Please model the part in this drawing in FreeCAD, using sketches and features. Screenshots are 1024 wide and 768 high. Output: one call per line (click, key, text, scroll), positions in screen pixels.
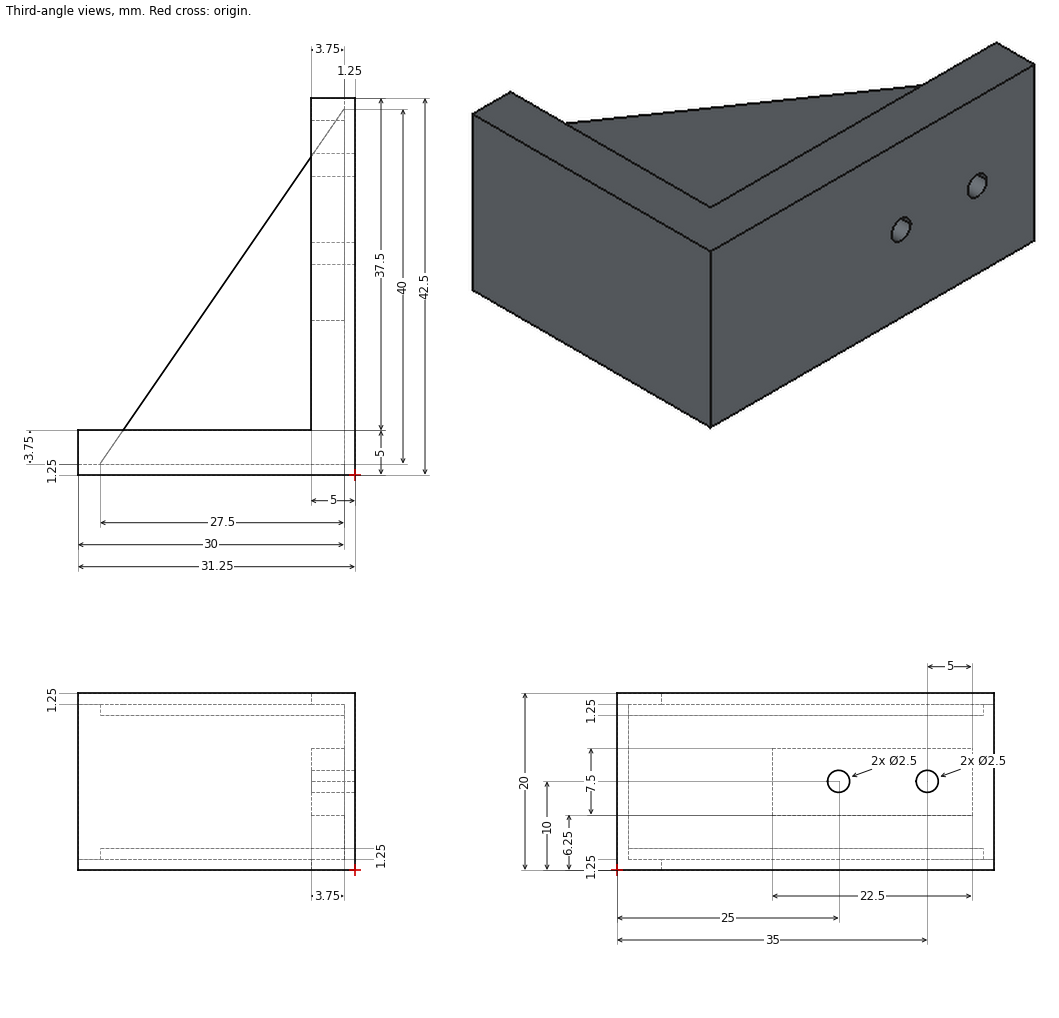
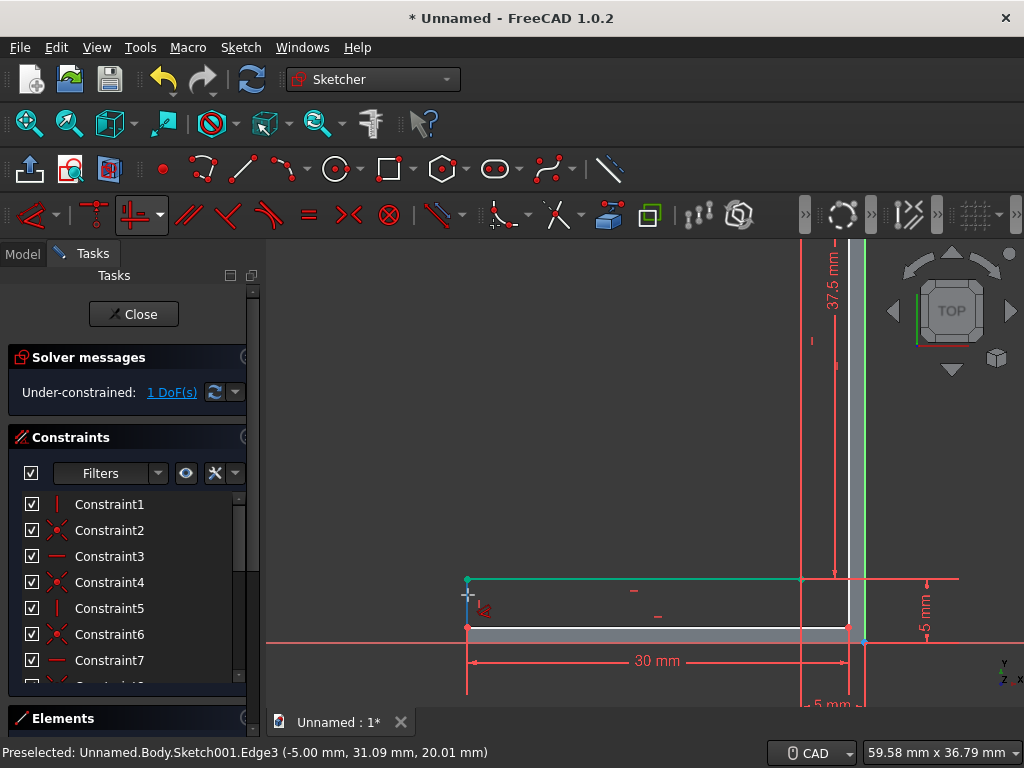
click(467, 594)
click(433, 604)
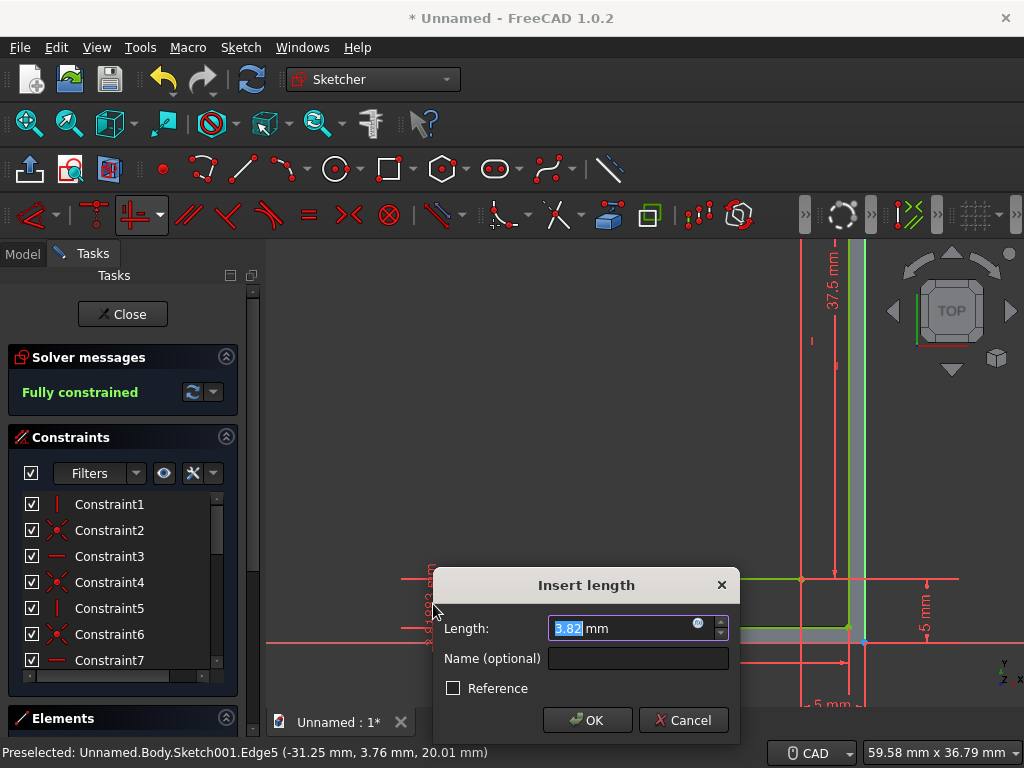
text(3.75)
key(Return)
key(Escape)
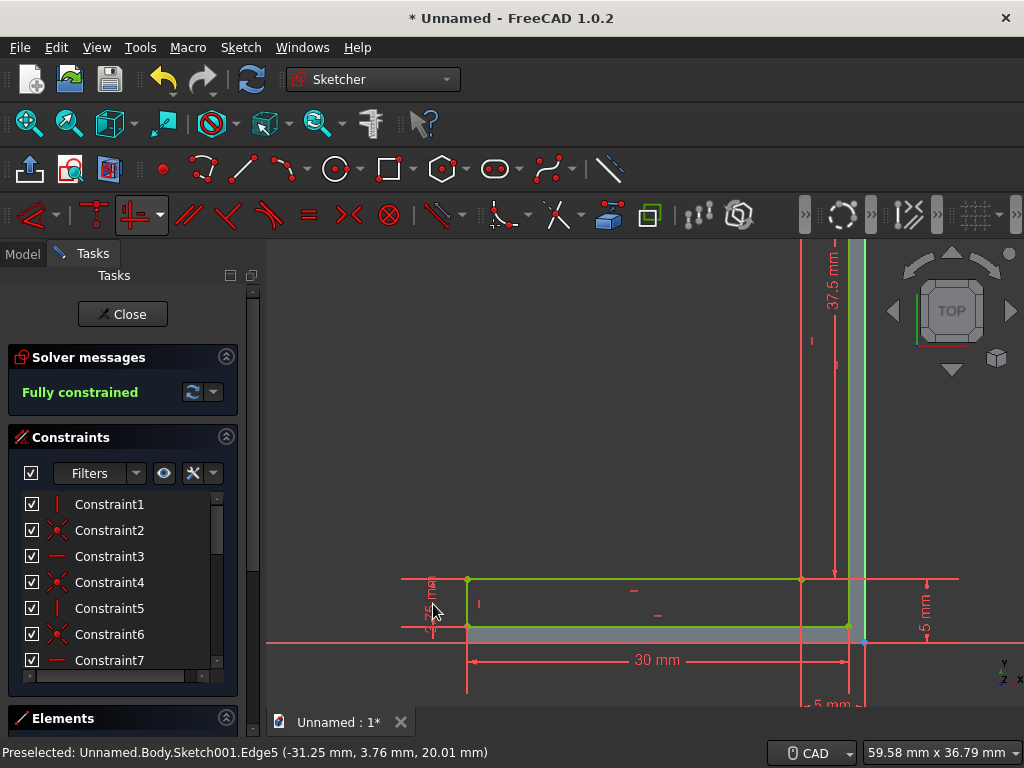
click(123, 314)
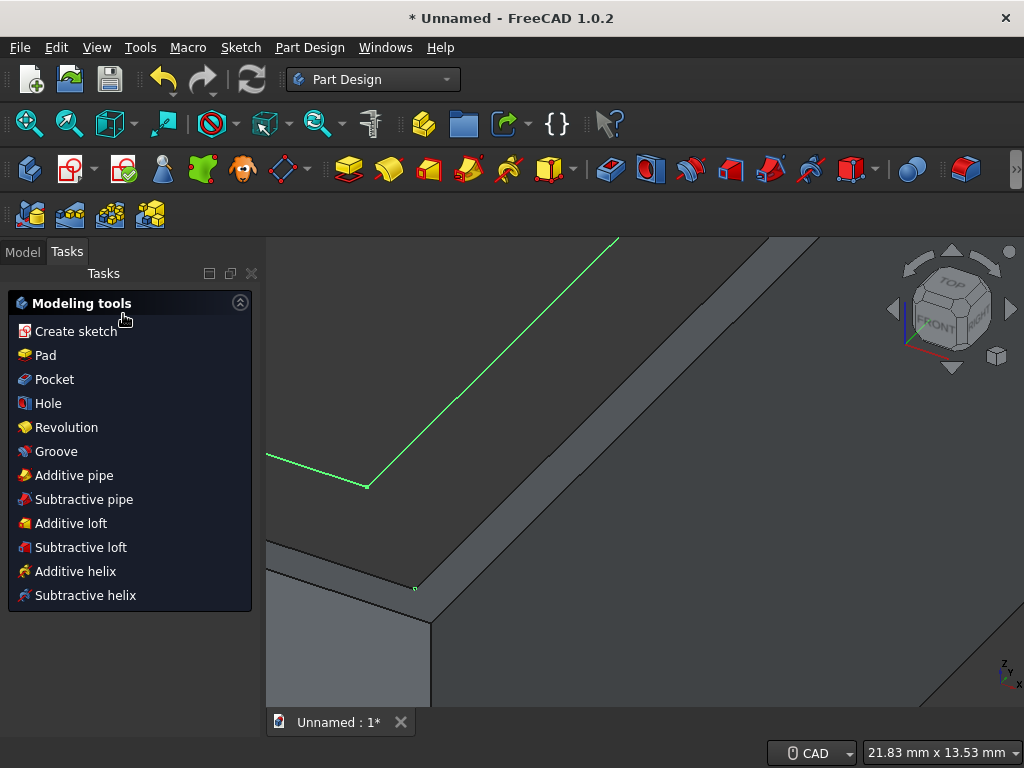
click(350, 170)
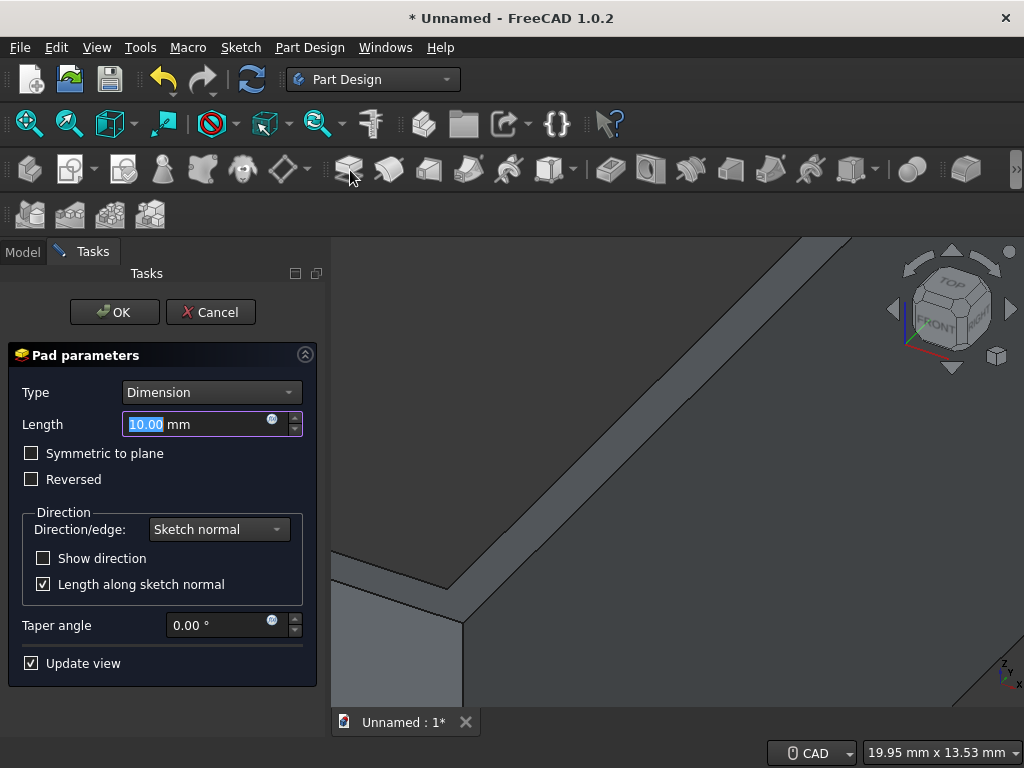
text(1.25)
key(Tab)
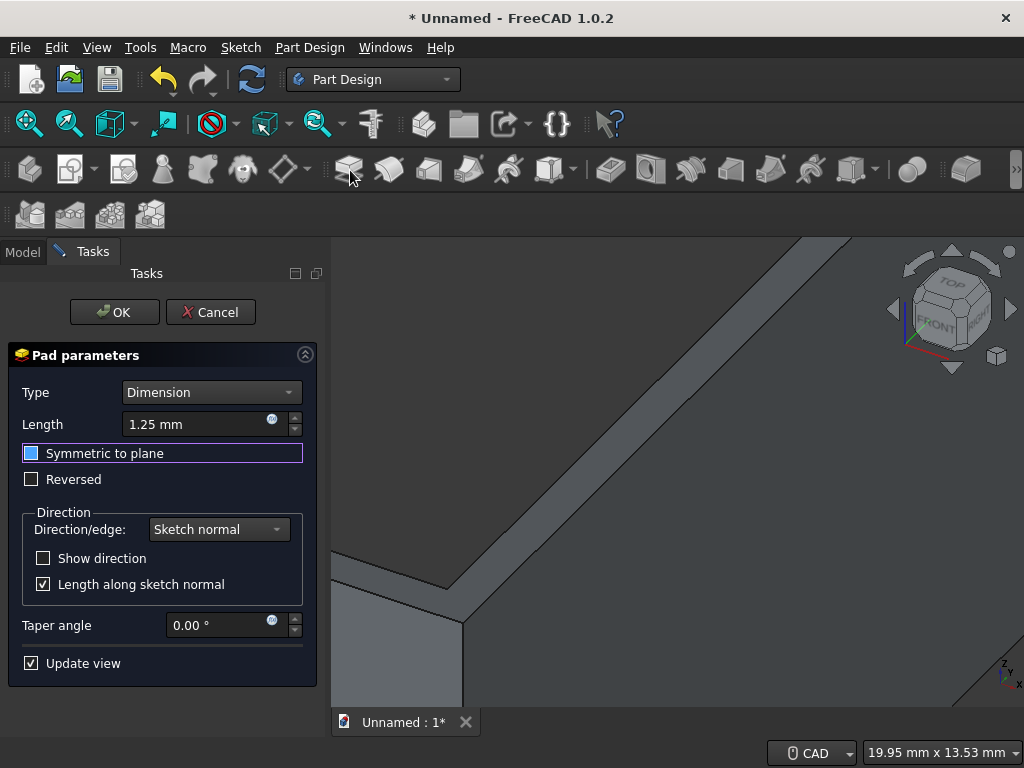
click(30, 479)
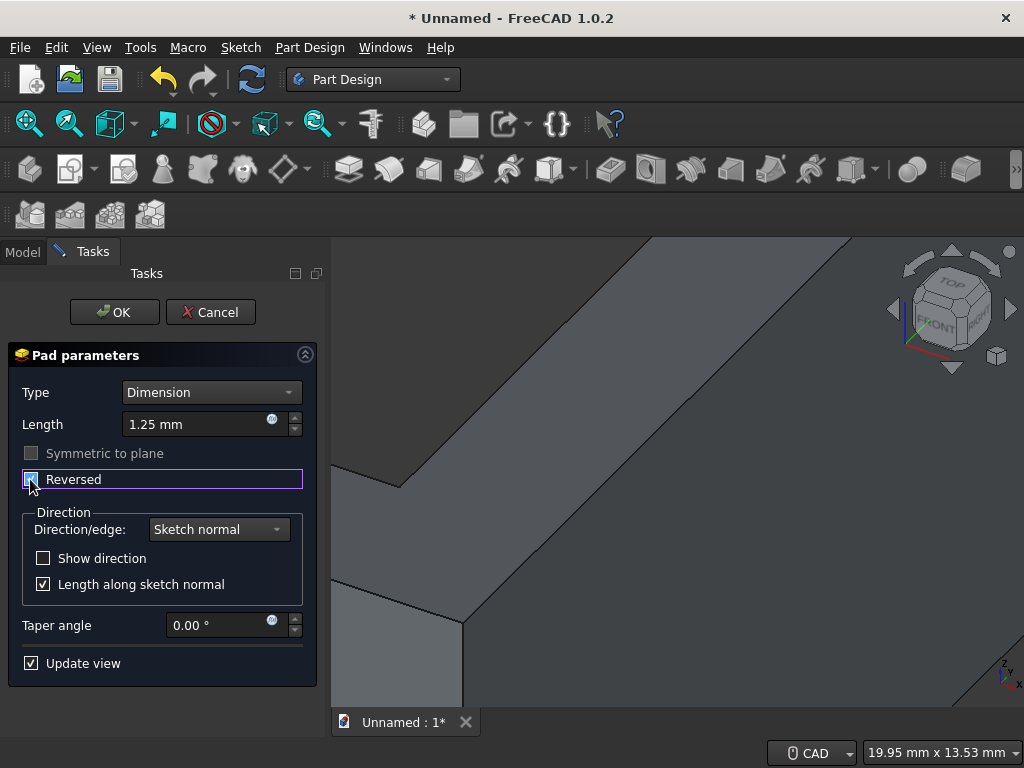
click(115, 312)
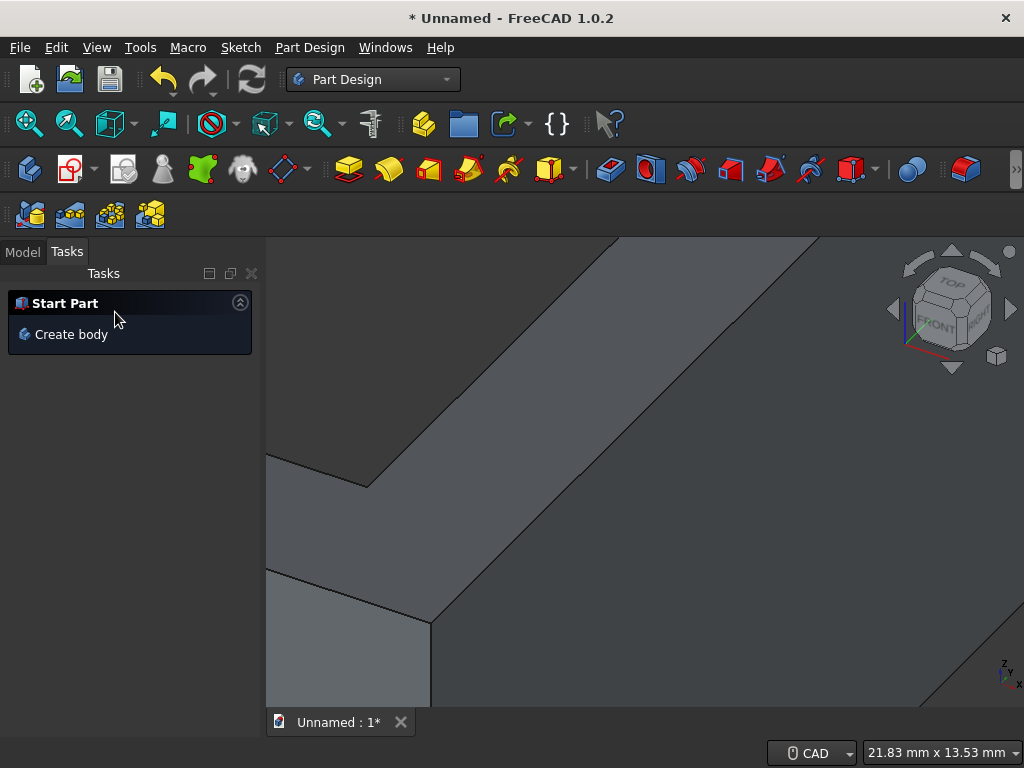
click(30, 124)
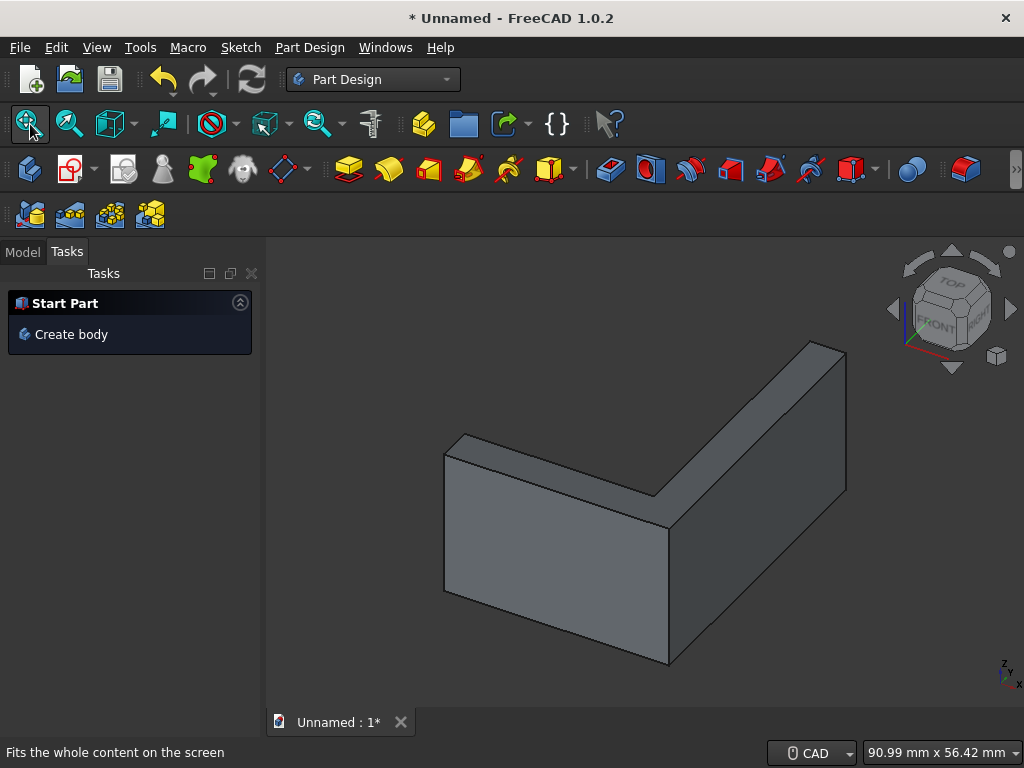
key(5)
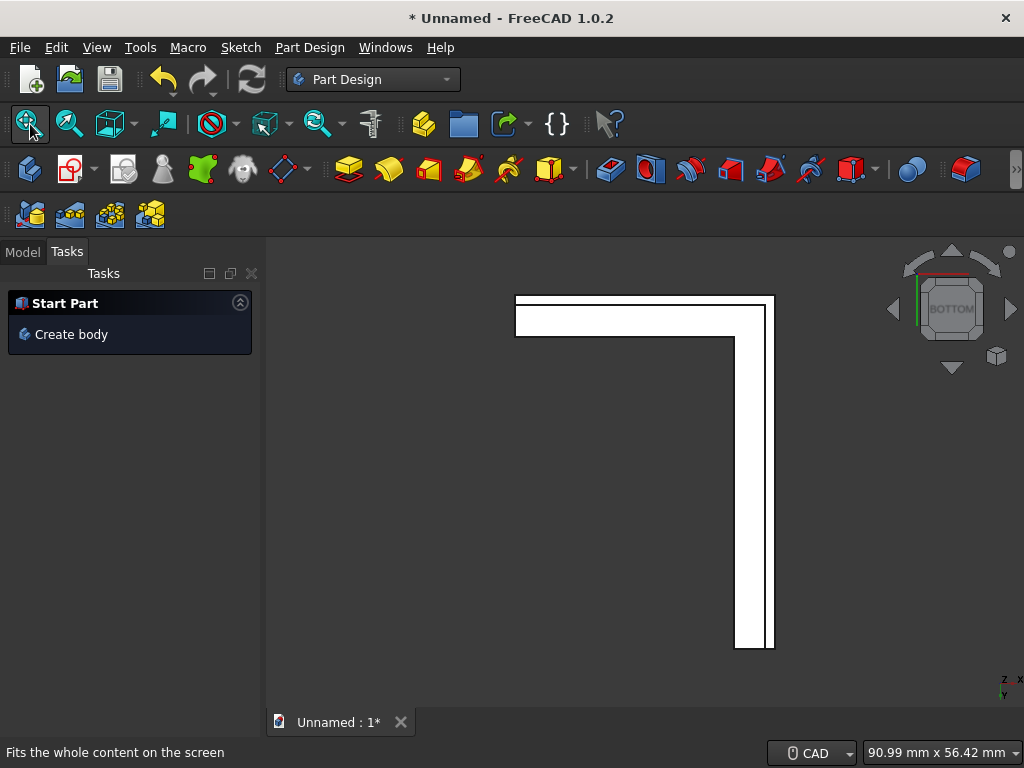
scroll(772, 415, up, 7)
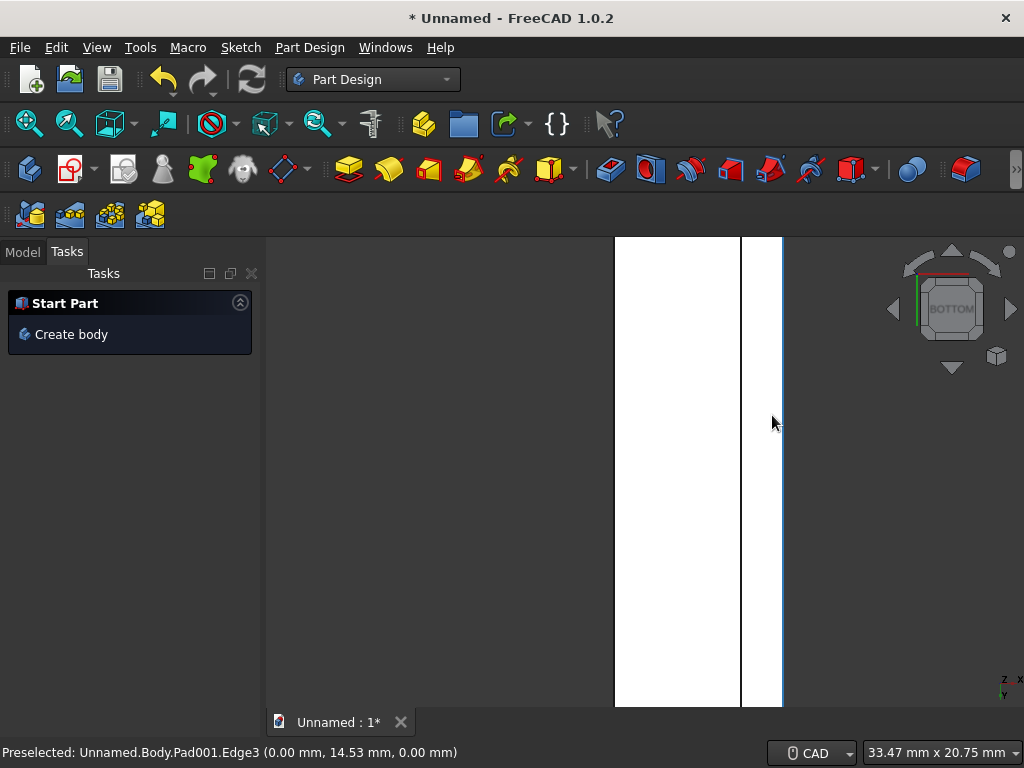
click(769, 419)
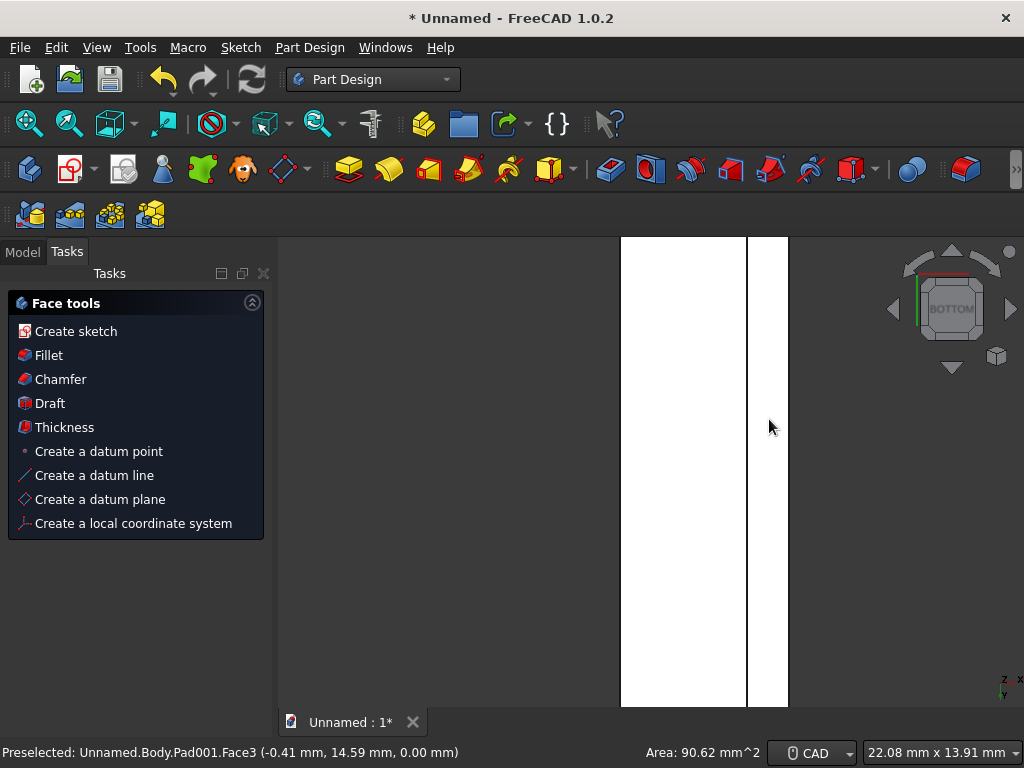
click(70, 170)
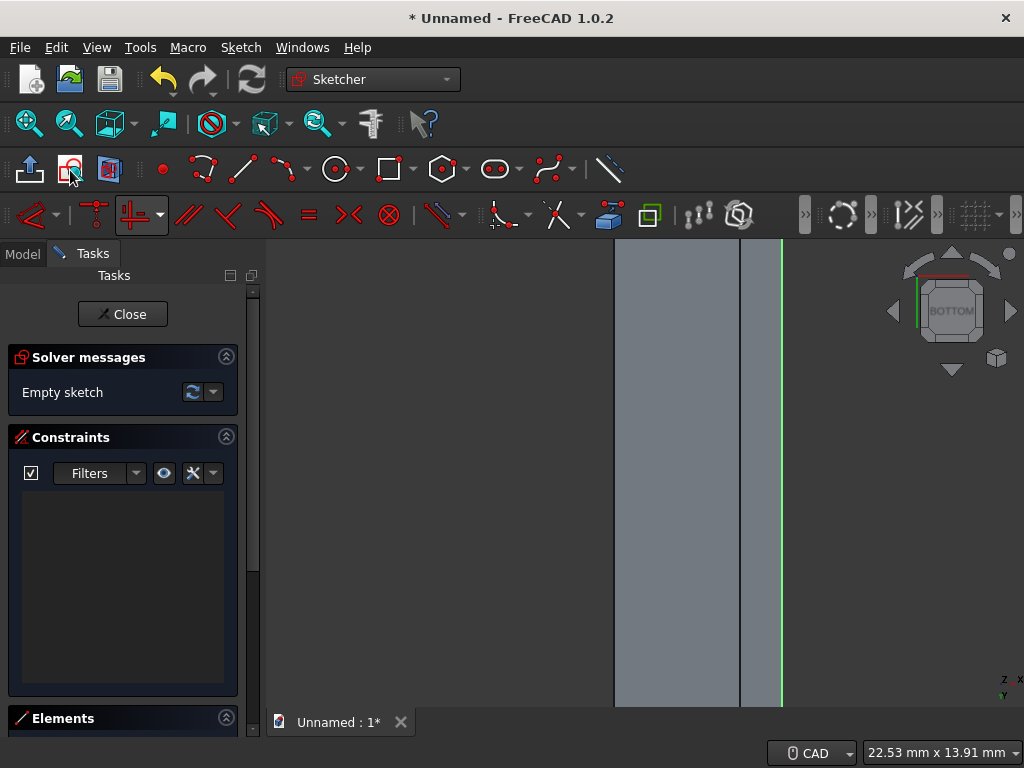
scroll(657, 429, down, 8)